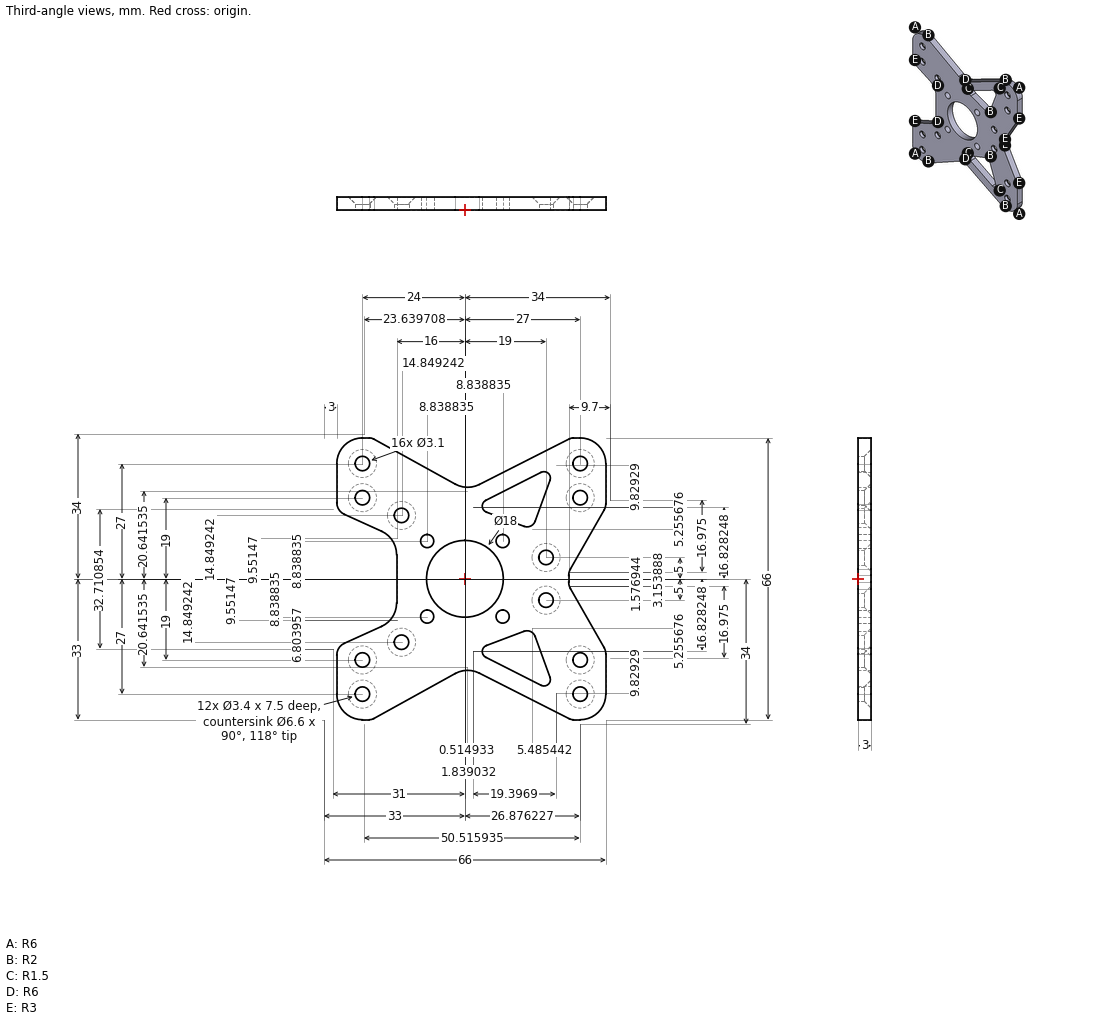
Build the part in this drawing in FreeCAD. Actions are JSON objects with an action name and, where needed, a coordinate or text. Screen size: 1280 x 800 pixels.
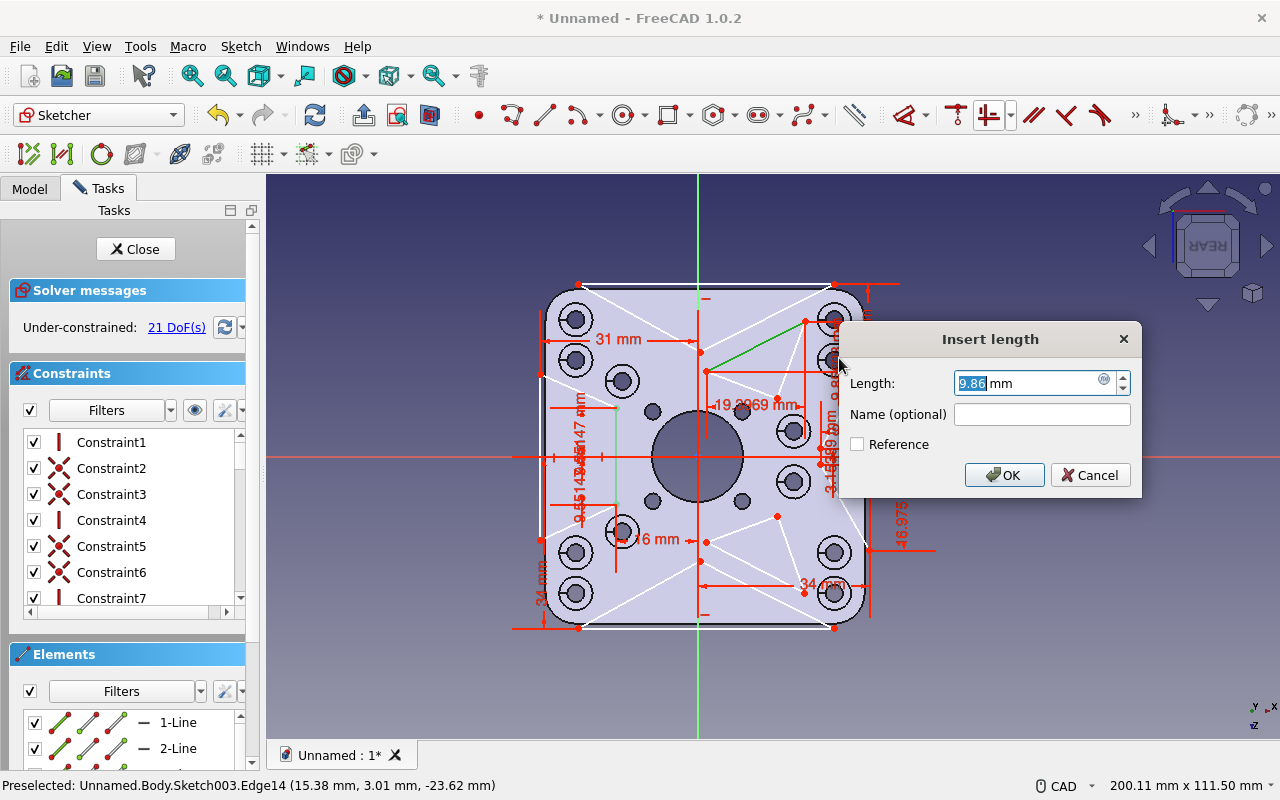
{"action": "type", "text": "9.82929"}
{"action": "key", "text": "Return"}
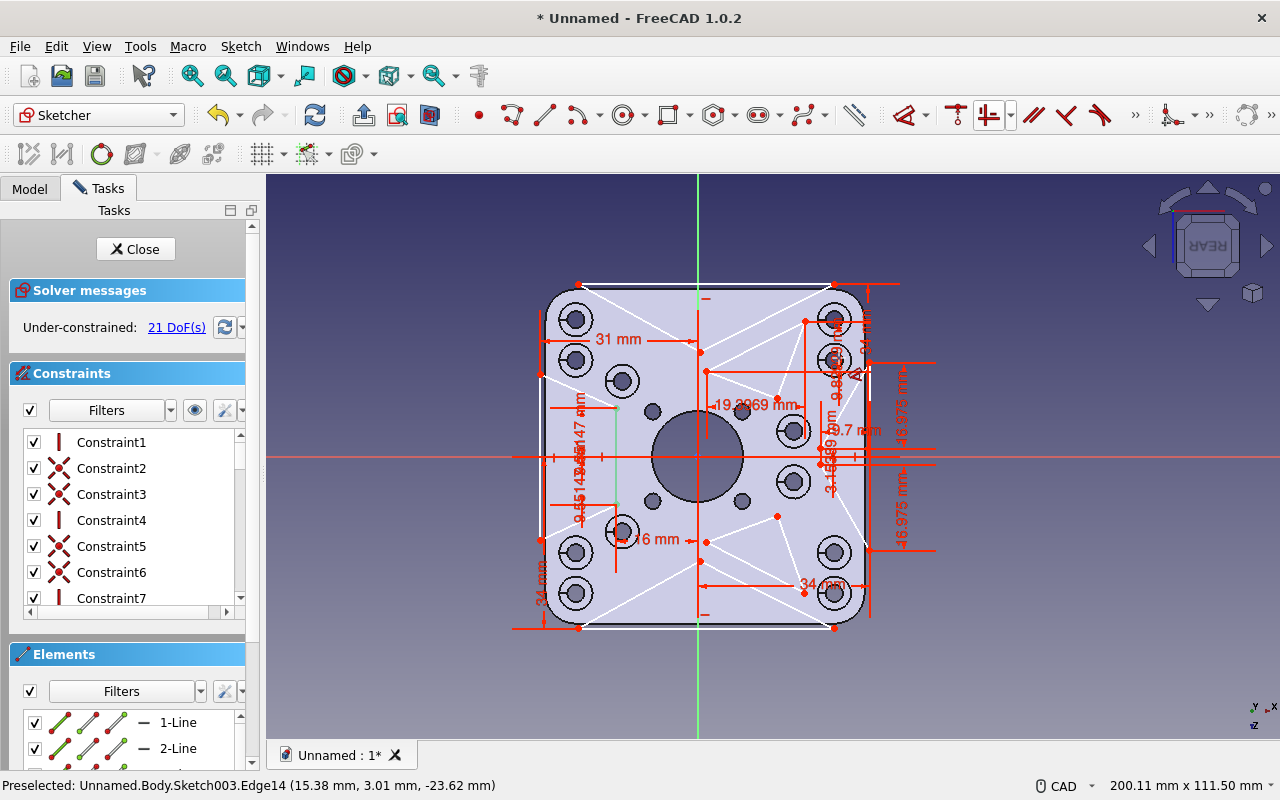
{"action": "left_click", "coordinate": [736, 558]}
{"action": "left_click", "coordinate": [756, 508]}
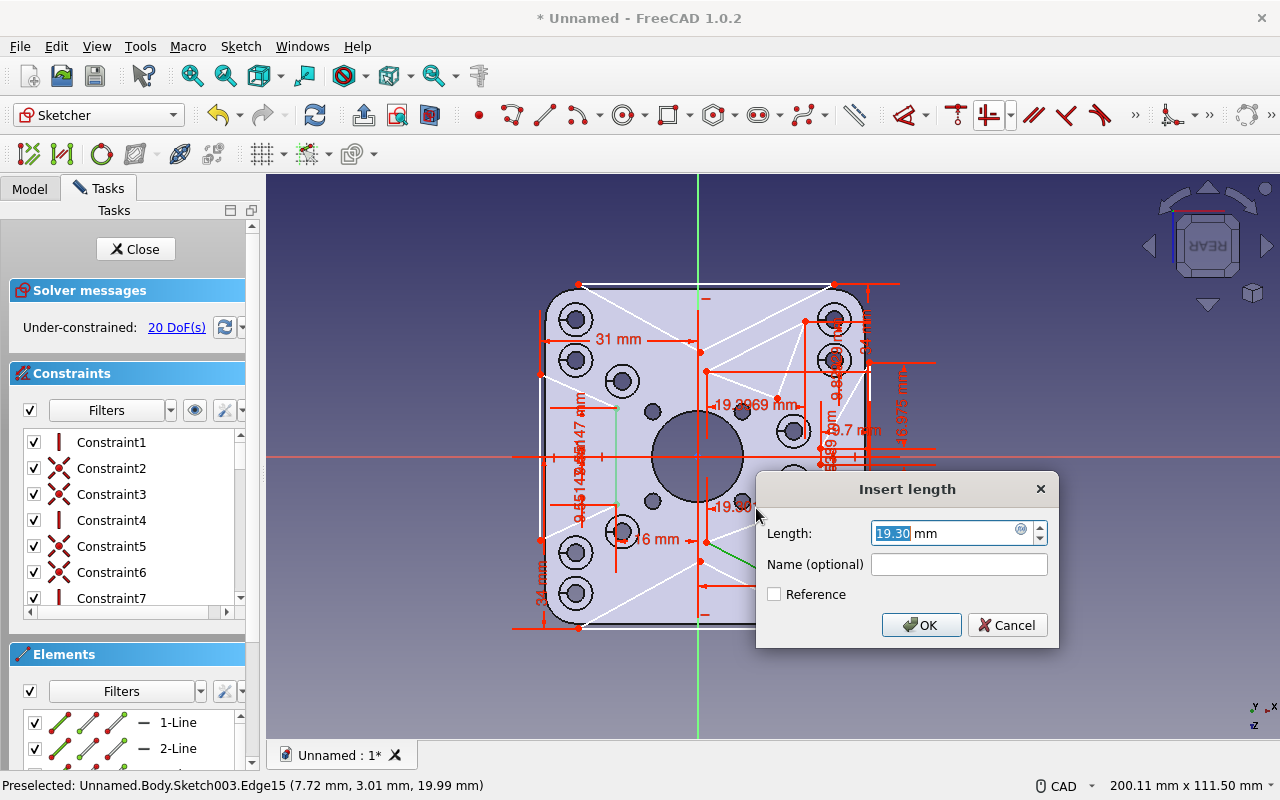
{"action": "type", "text": "19.3969"}
{"action": "key", "text": "Return"}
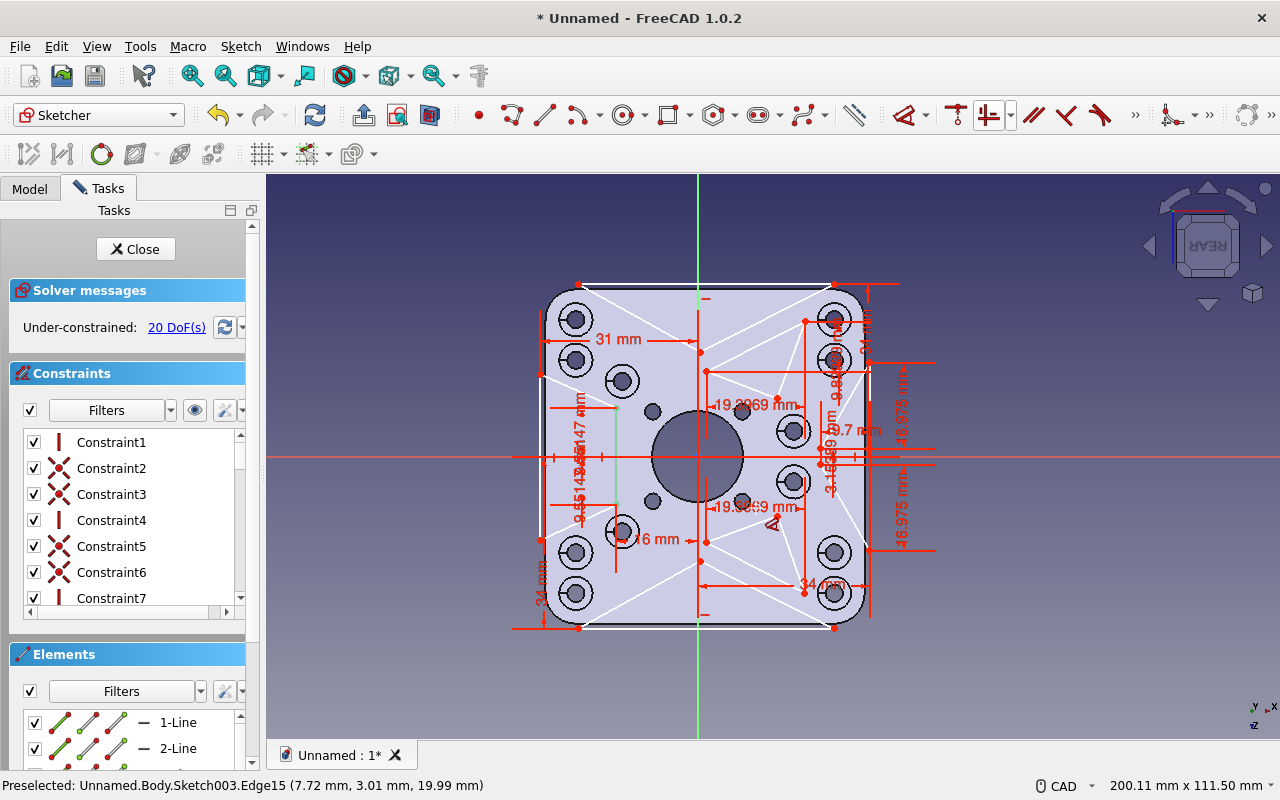
{"action": "left_click", "coordinate": [736, 558]}
{"action": "left_click", "coordinate": [839, 556]}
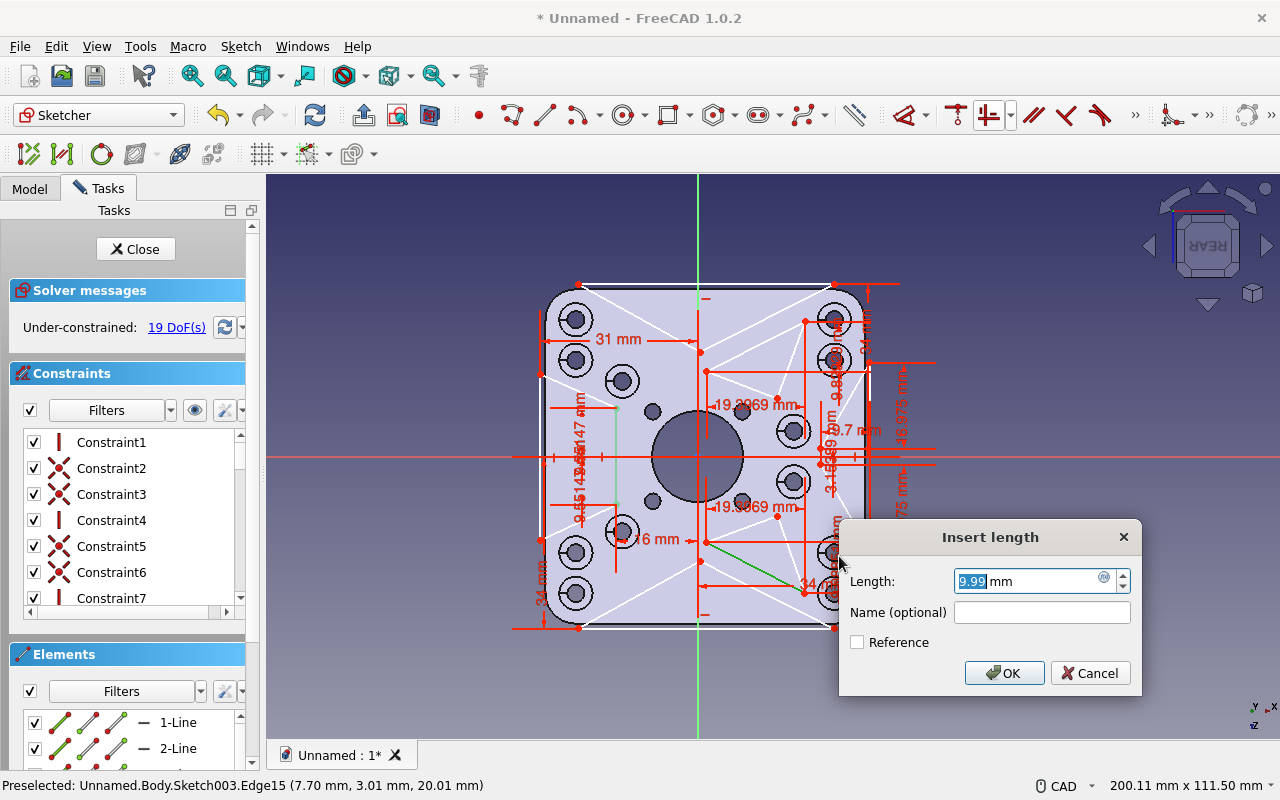
{"action": "type", "text": "9.82929"}
{"action": "key", "text": "Return"}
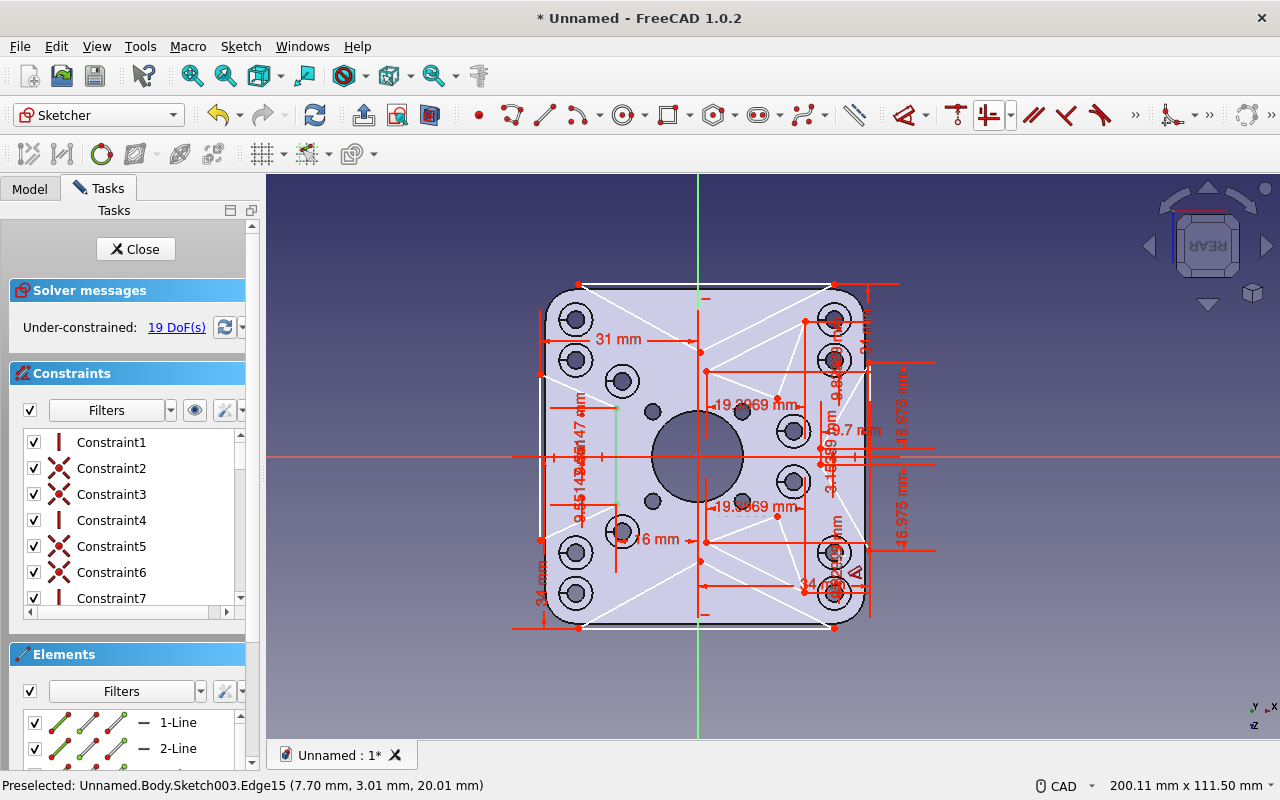
{"action": "left_click", "coordinate": [540, 424]}
{"action": "left_click", "coordinate": [506, 419]}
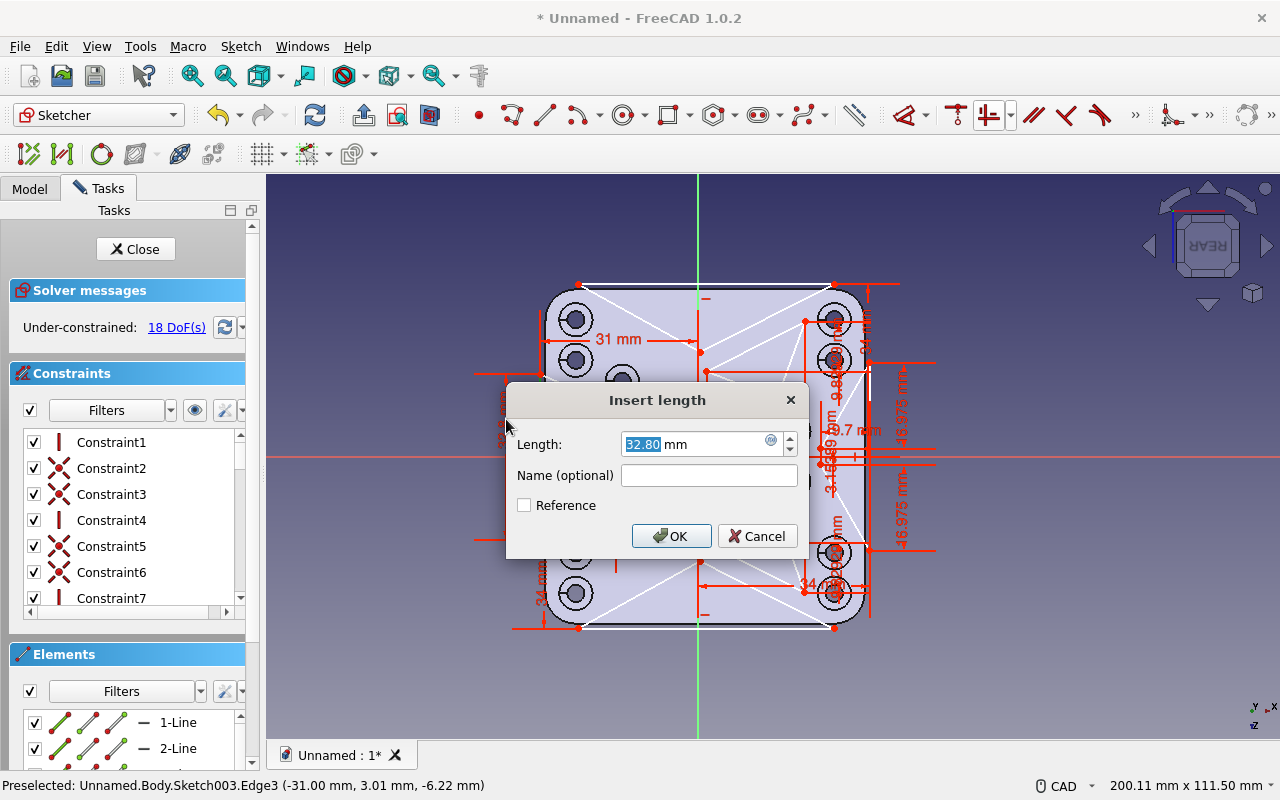
{"action": "type", "text": "32.710854"}
{"action": "key", "text": "Return"}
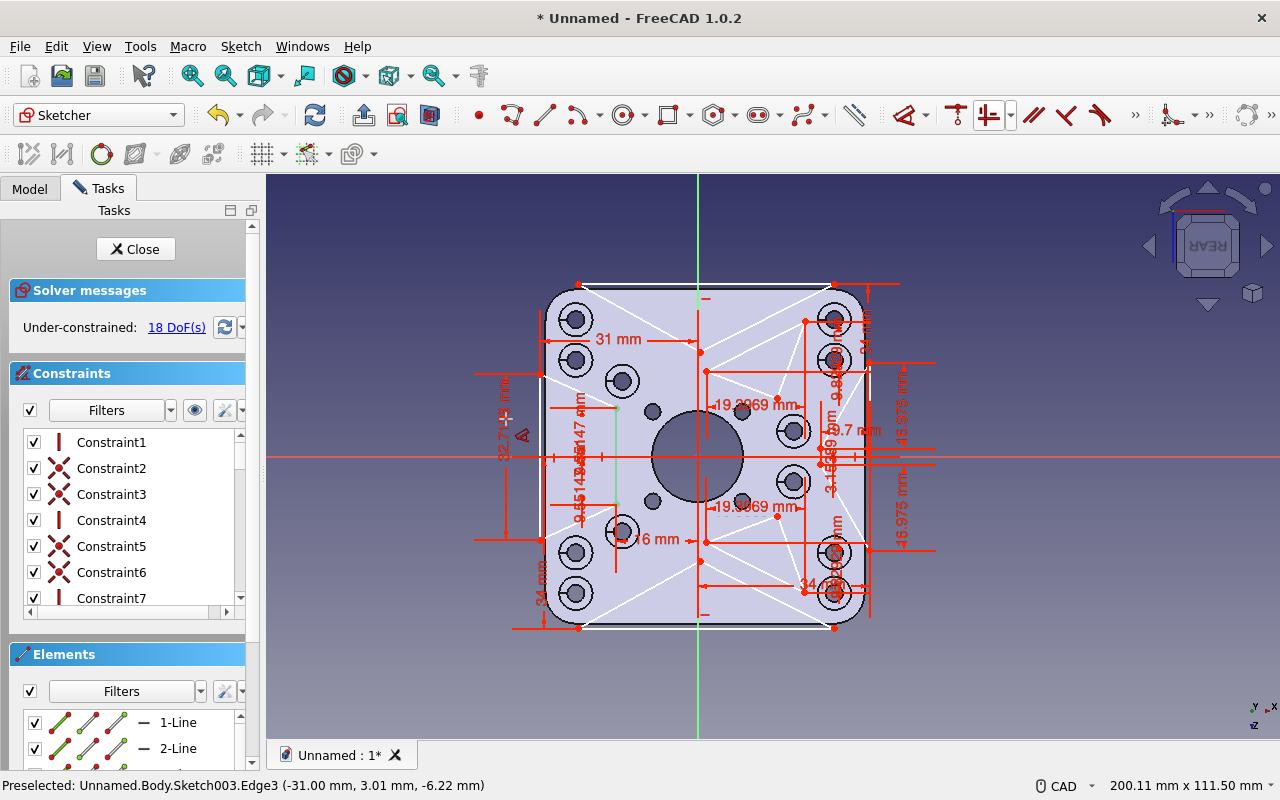
{"action": "left_click", "coordinate": [757, 284]}
{"action": "left_click", "coordinate": [647, 250]}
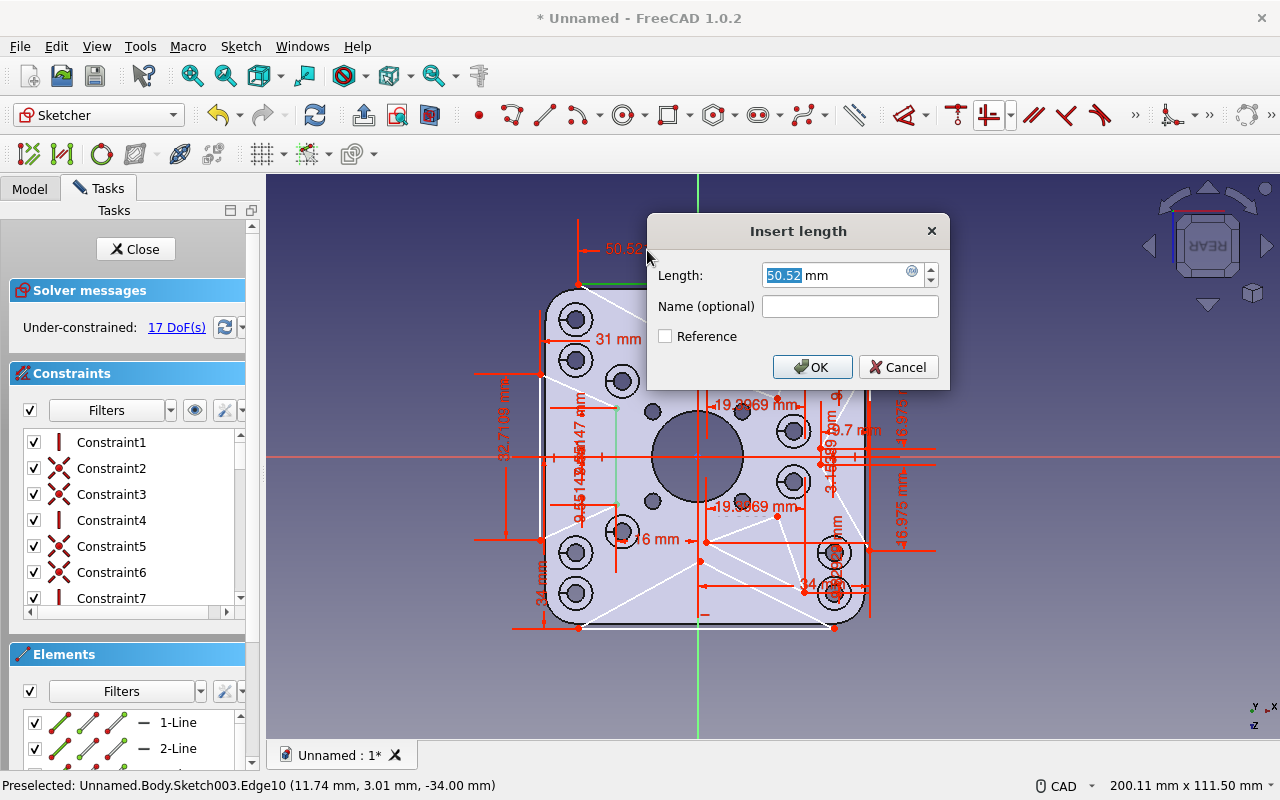
{"action": "type", "text": "50.515935"}
{"action": "key", "text": "Return"}